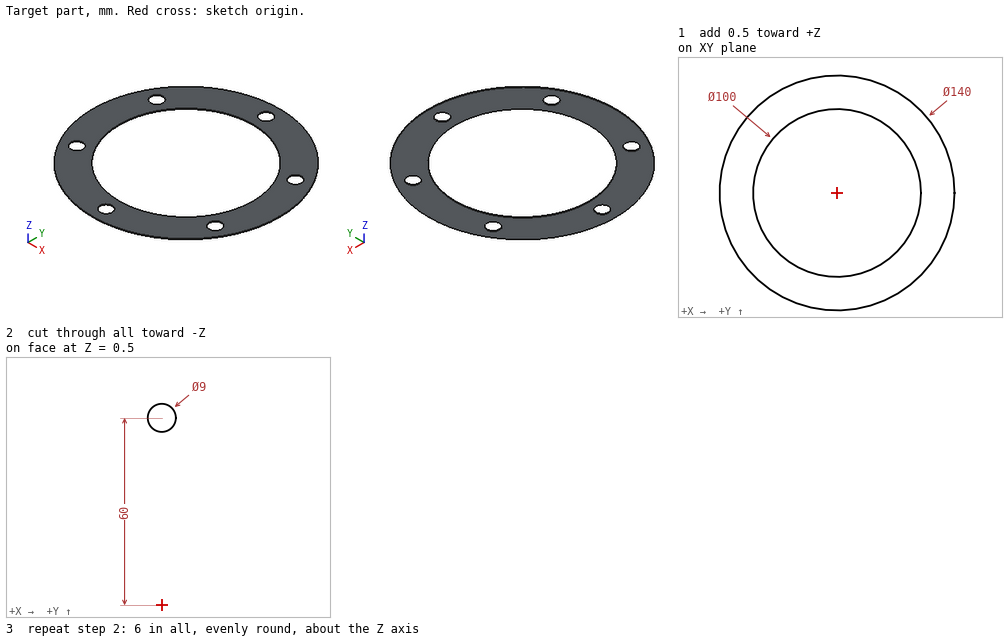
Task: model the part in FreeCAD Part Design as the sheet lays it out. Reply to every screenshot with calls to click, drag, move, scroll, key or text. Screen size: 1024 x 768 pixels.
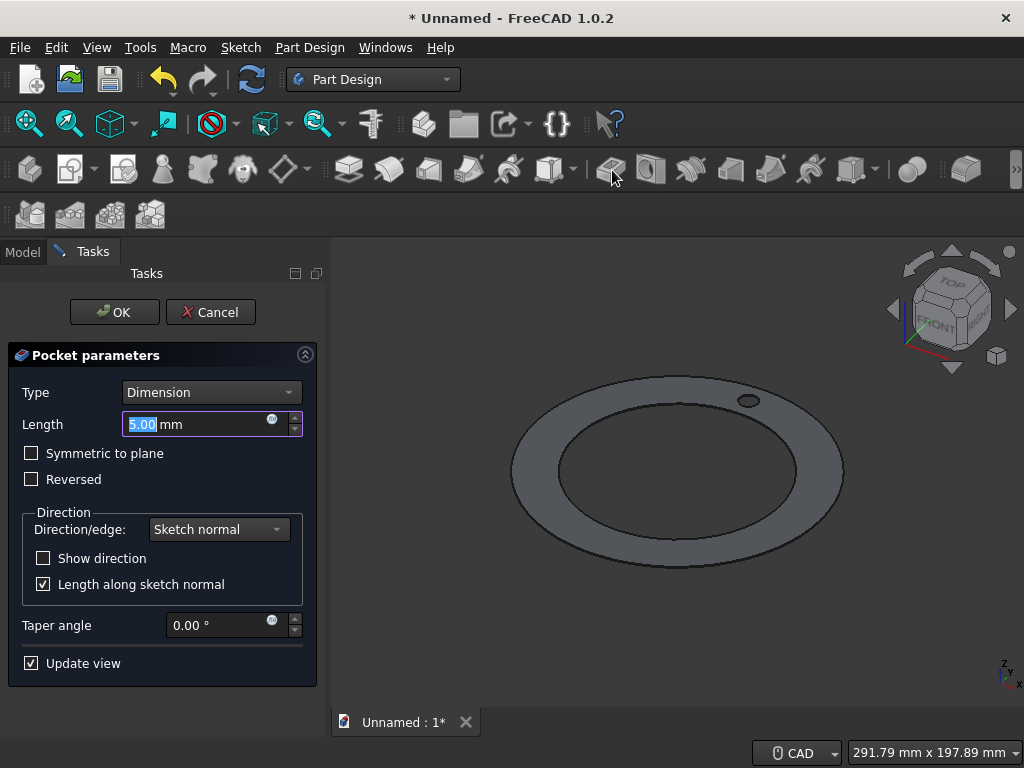
click(212, 392)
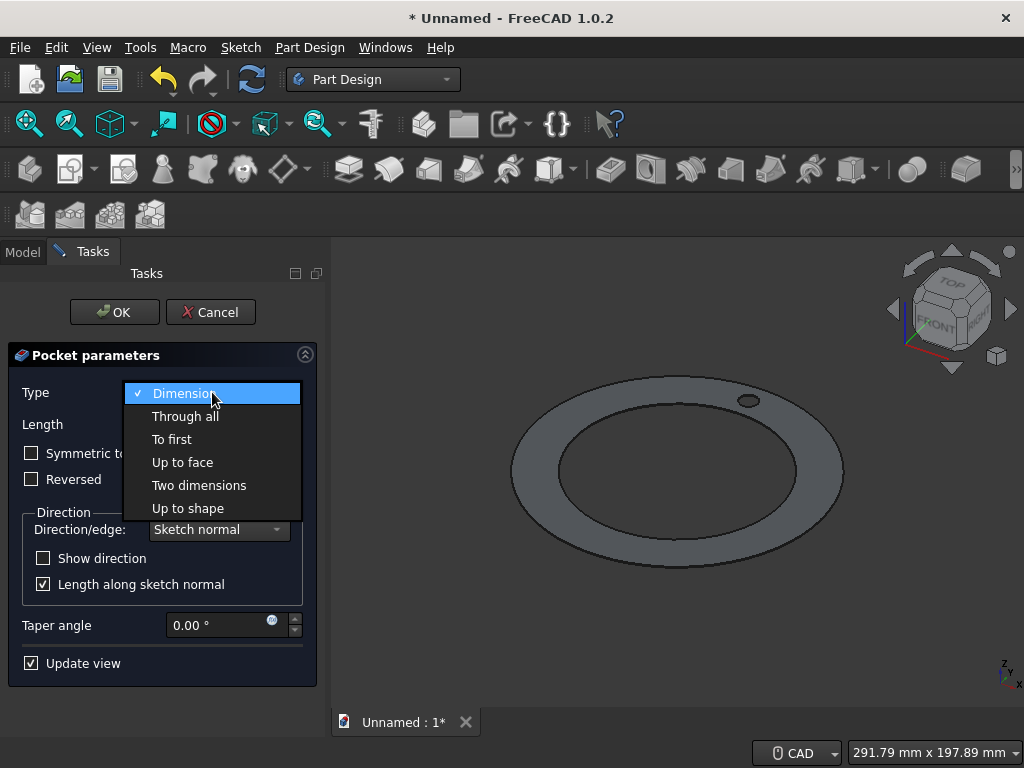
click(212, 416)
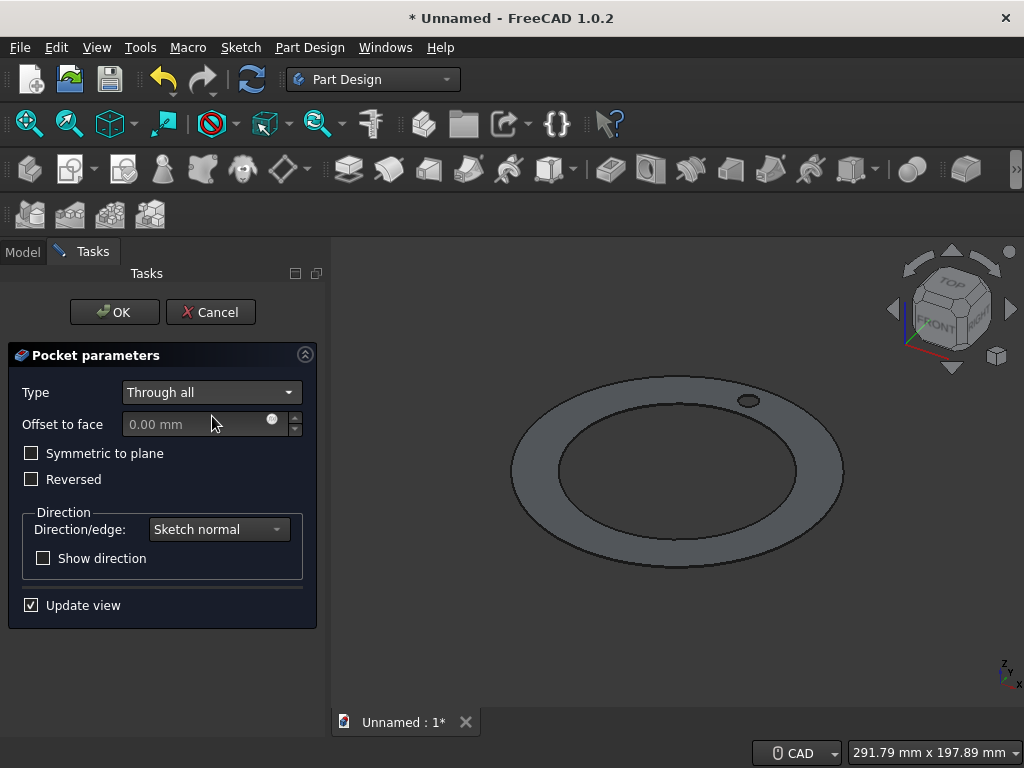
click(115, 312)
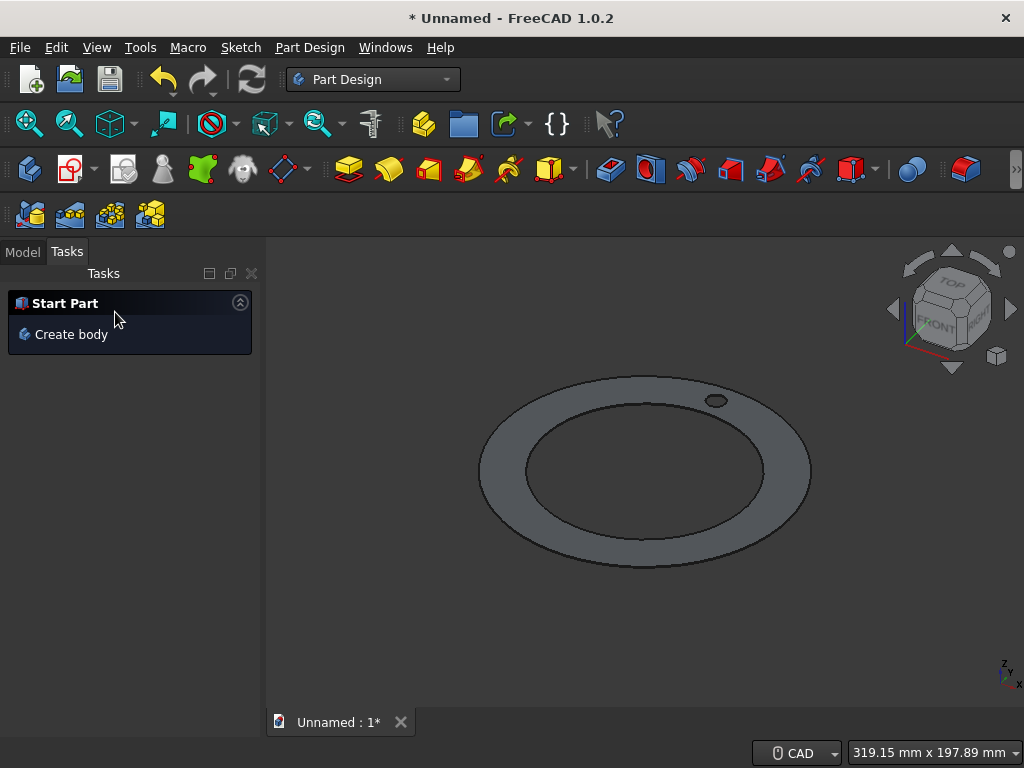
click(23, 251)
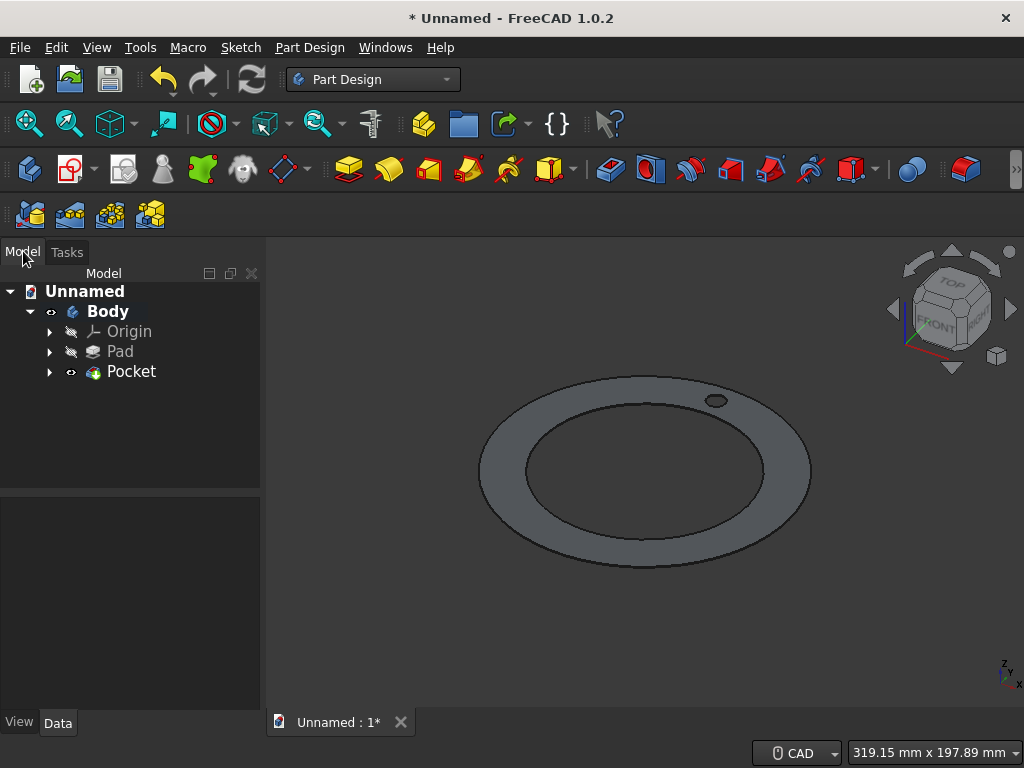
click(116, 372)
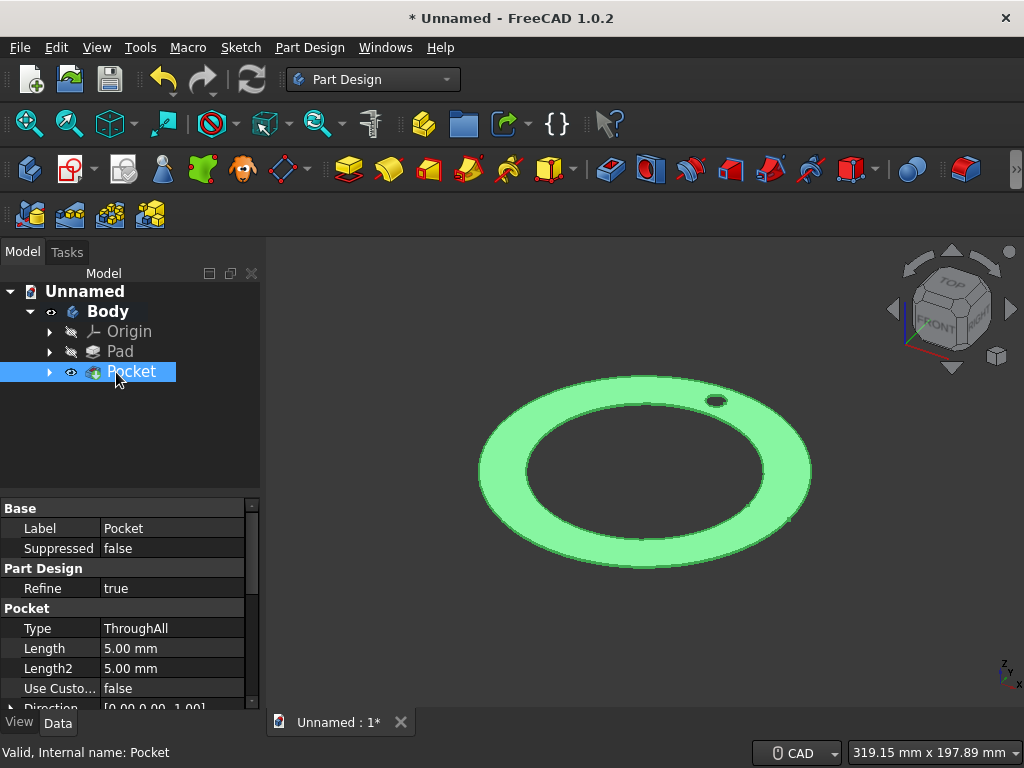
click(110, 214)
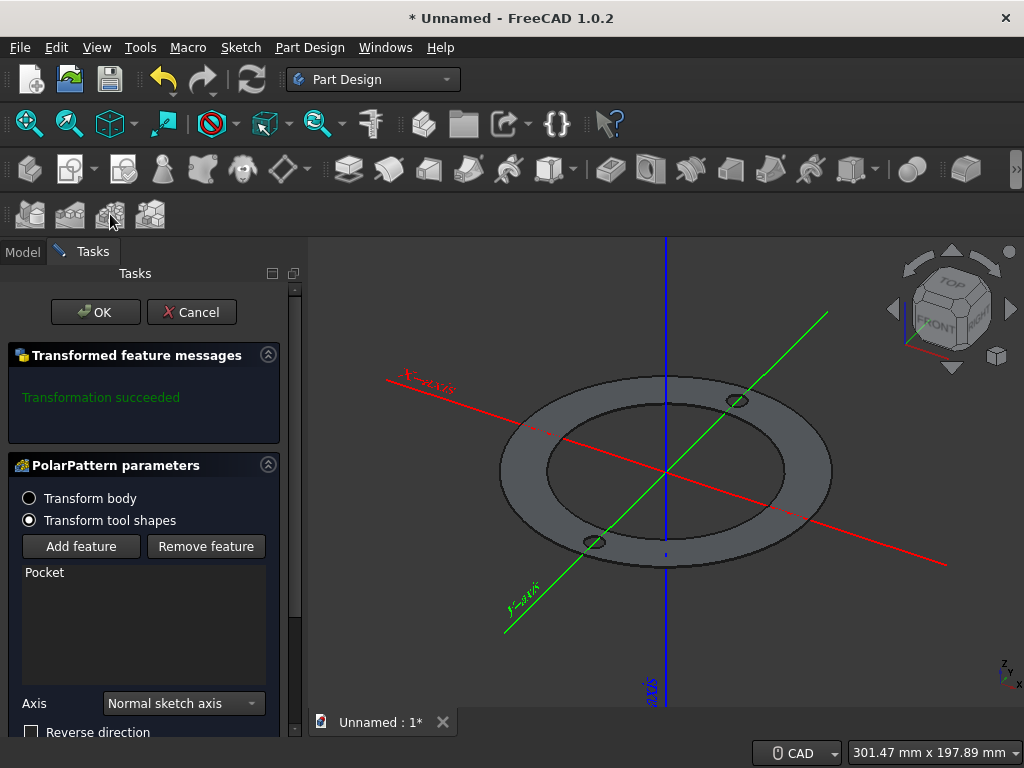
click(184, 704)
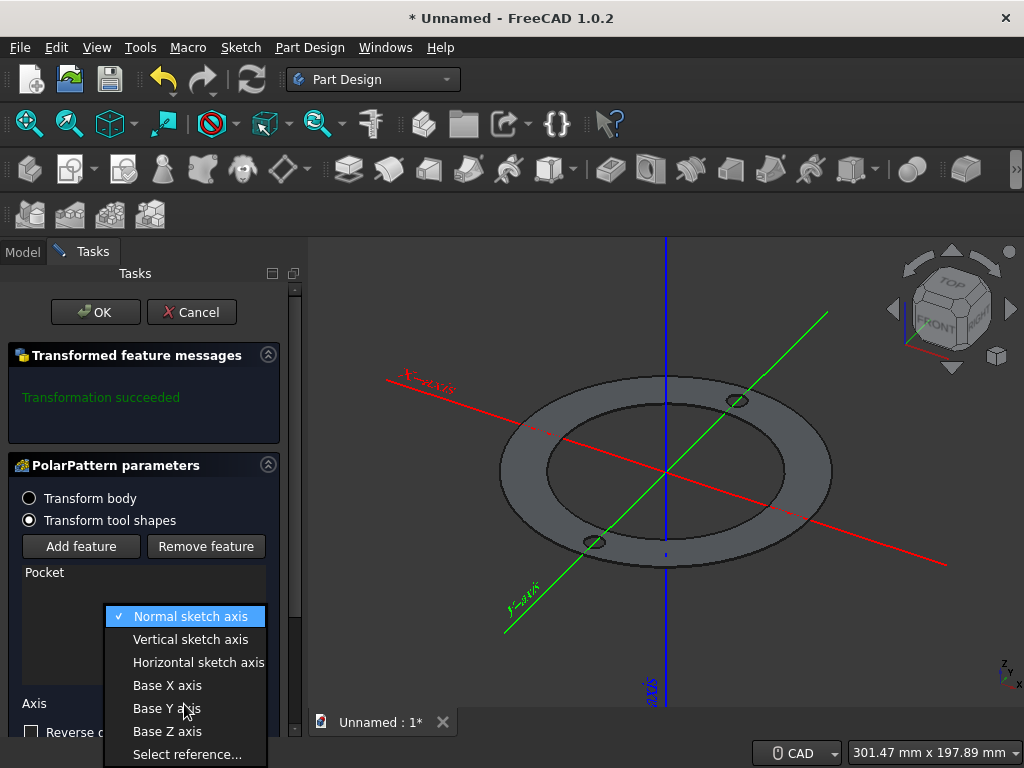
click(184, 732)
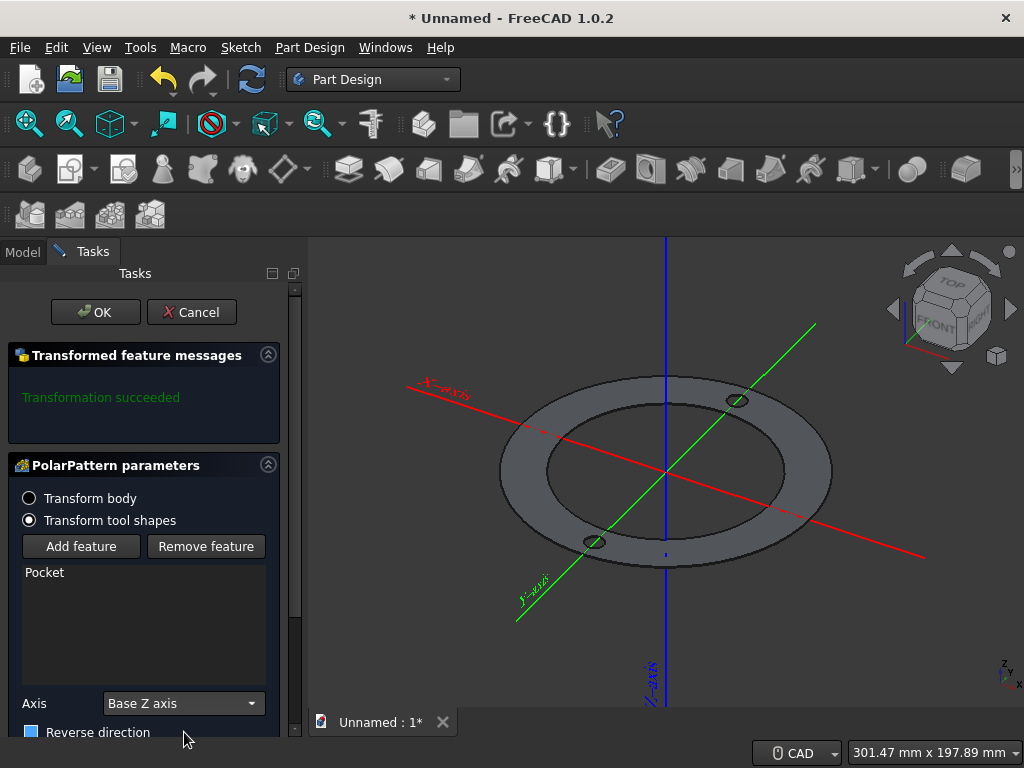
scroll(295, 510, down, 3)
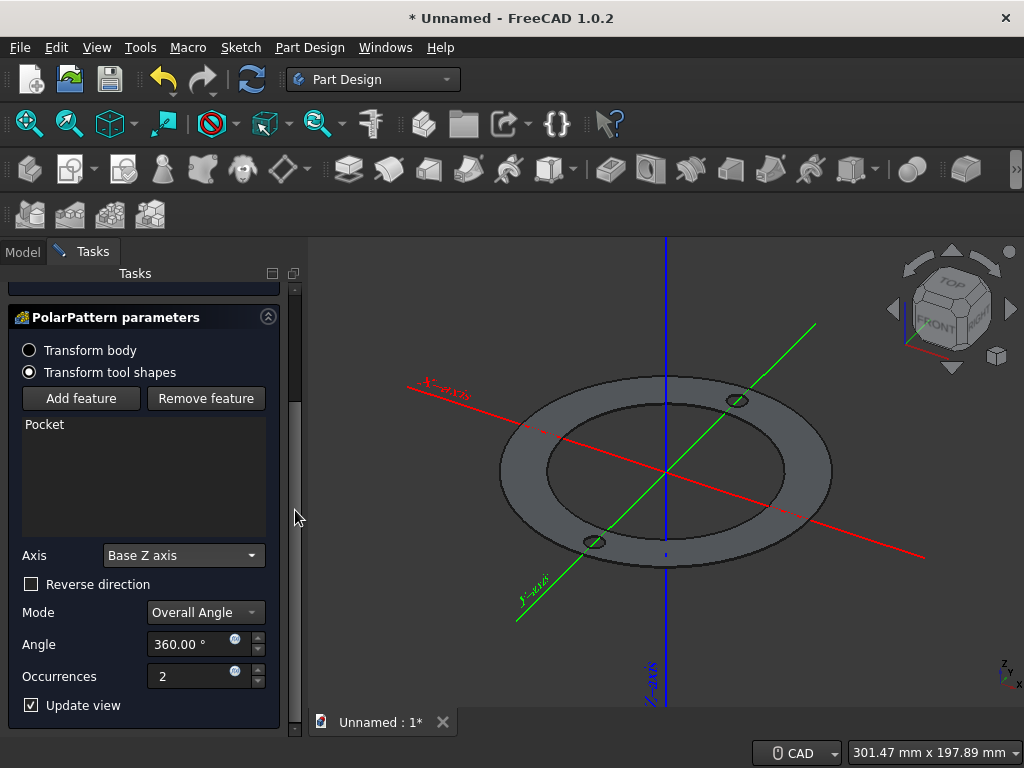
triple_click(198, 676)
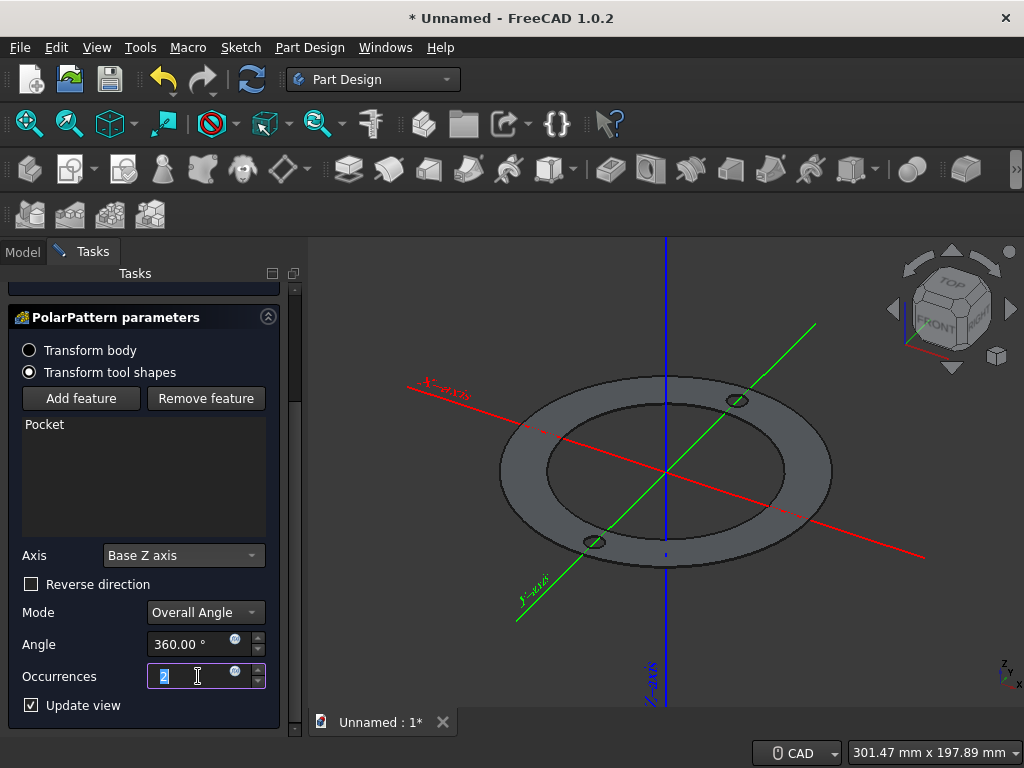
text(6)
key(Tab)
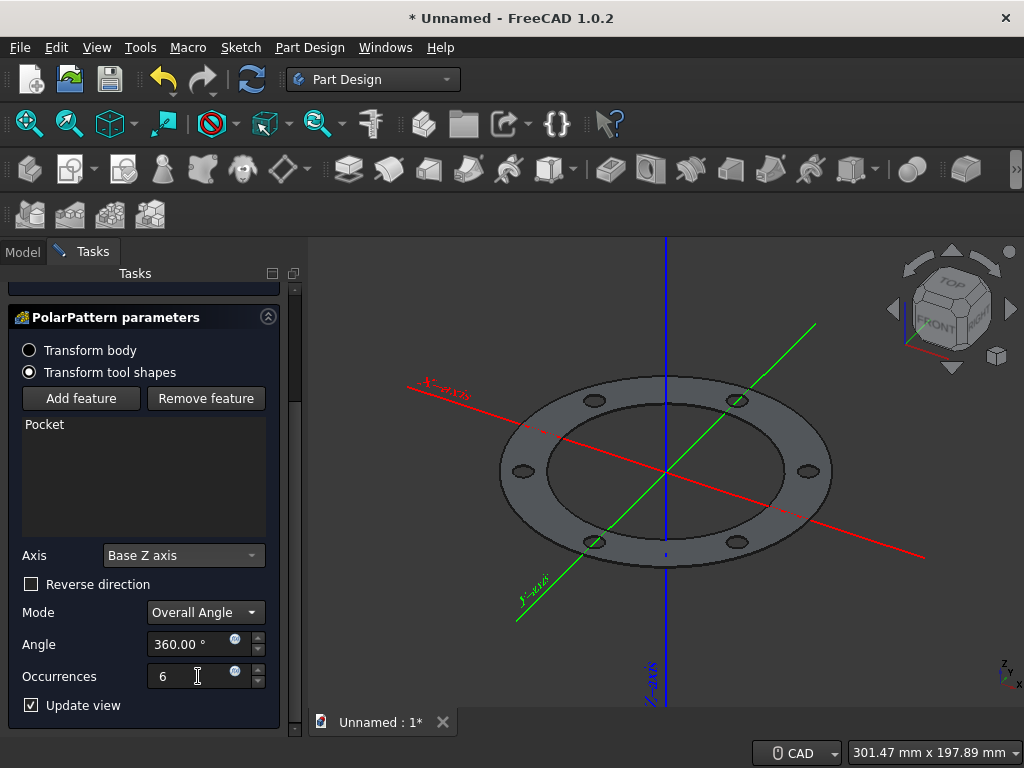
scroll(295, 510, up, 4)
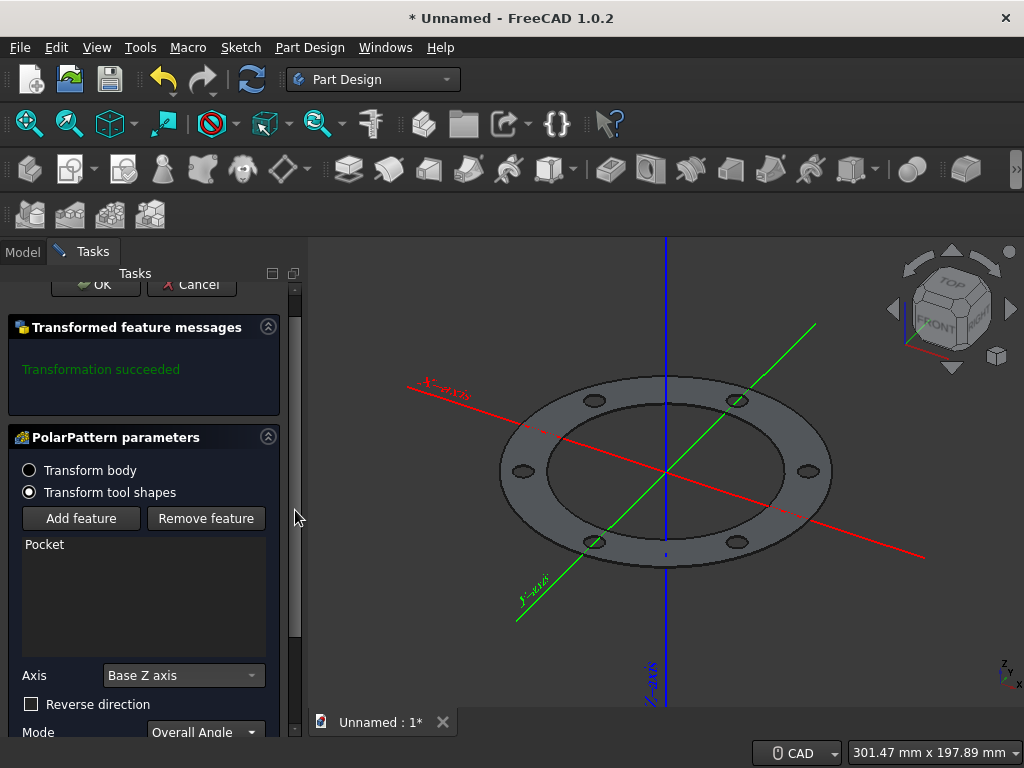
click(96, 312)